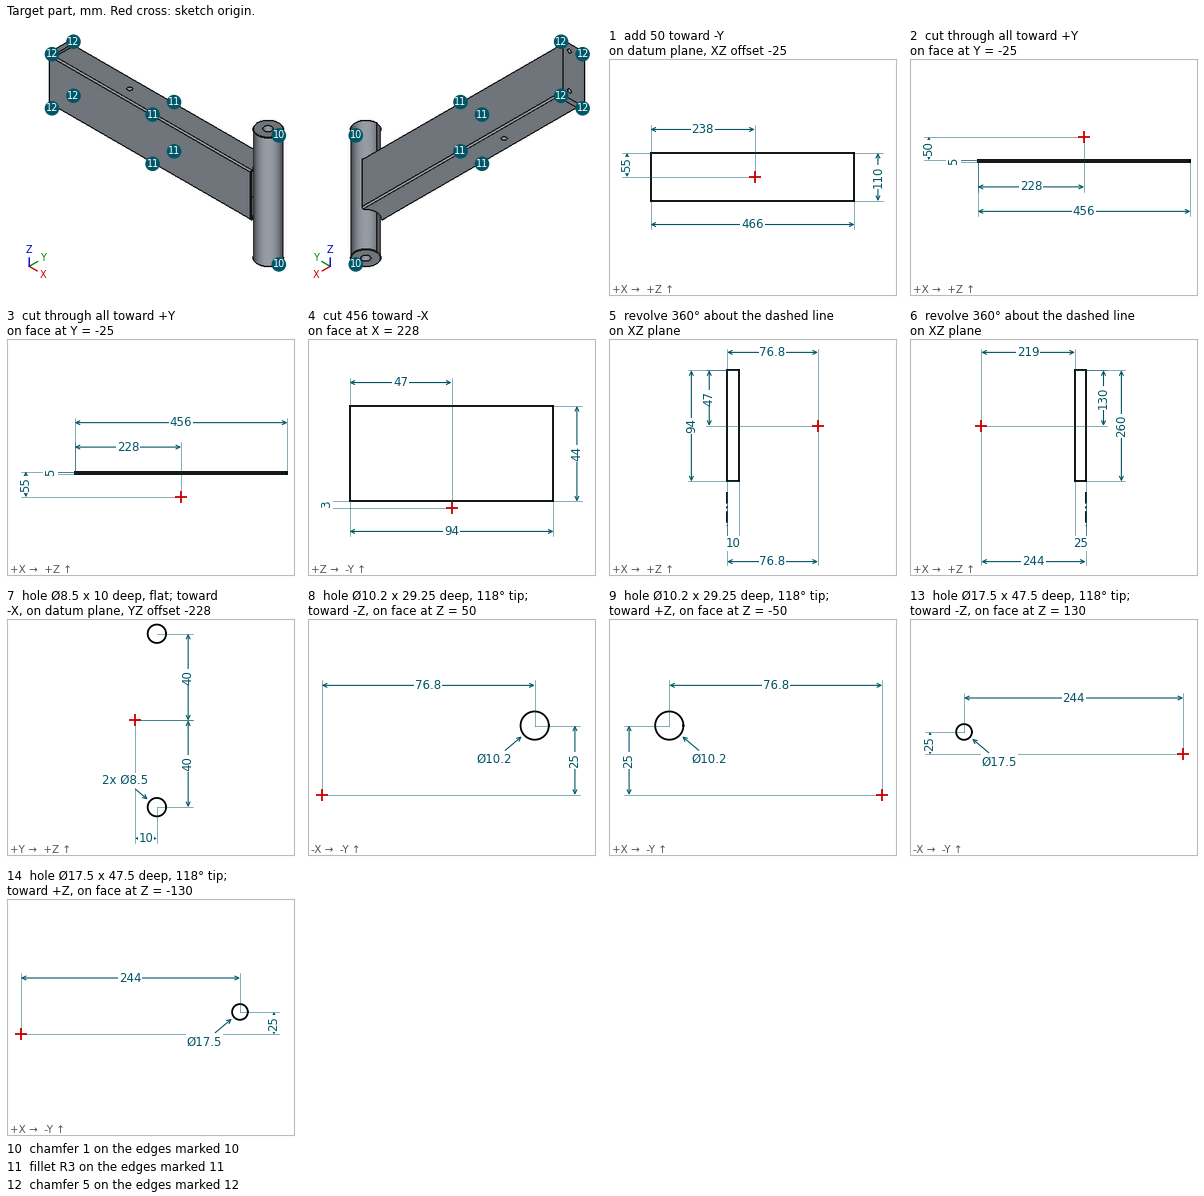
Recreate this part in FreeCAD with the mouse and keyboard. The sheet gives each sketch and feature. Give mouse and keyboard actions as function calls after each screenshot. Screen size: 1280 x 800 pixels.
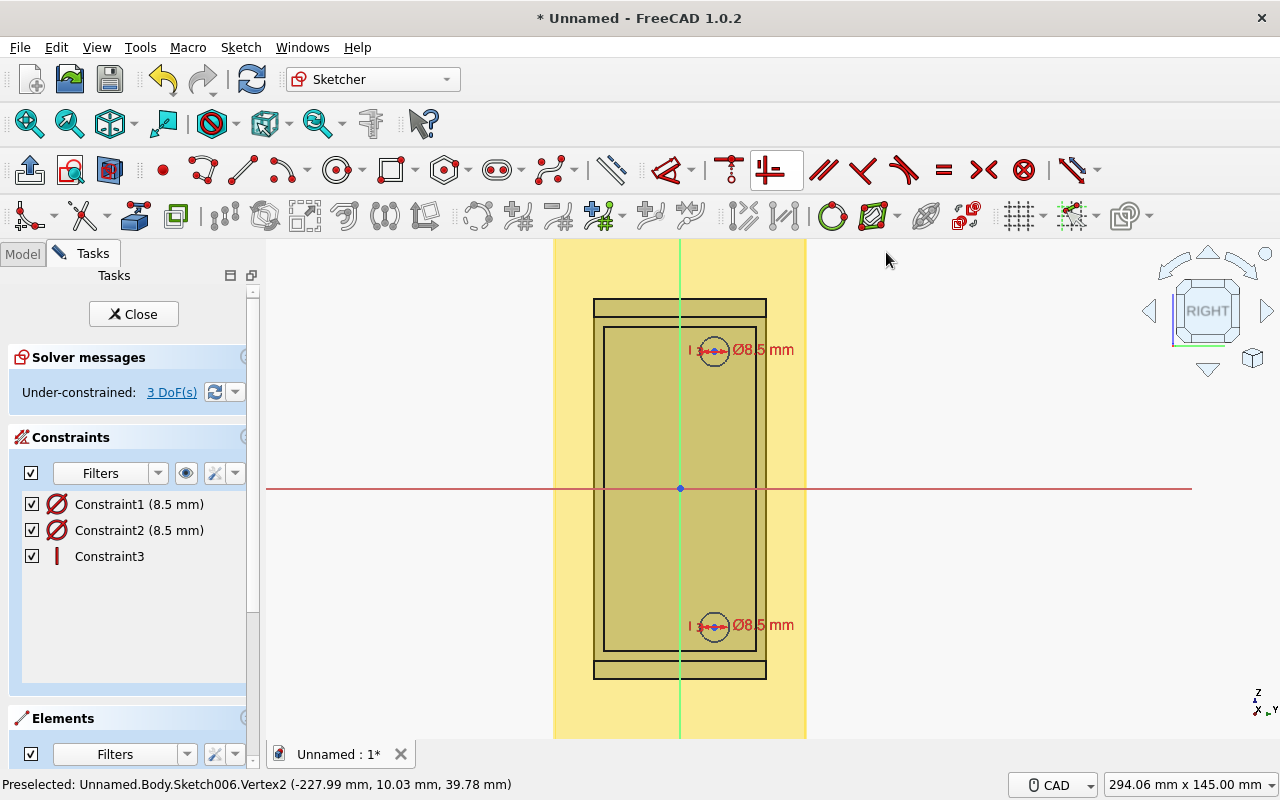
click(666, 170)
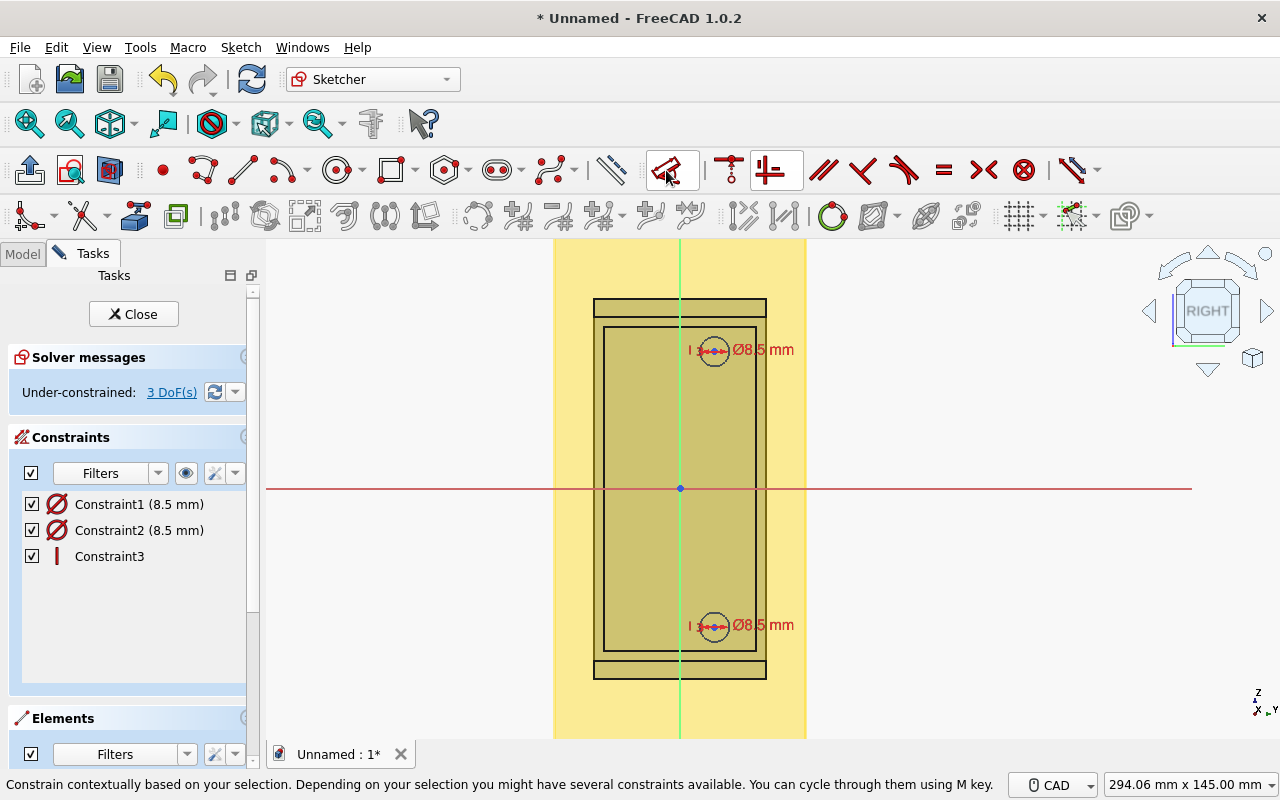
click(715, 627)
click(697, 661)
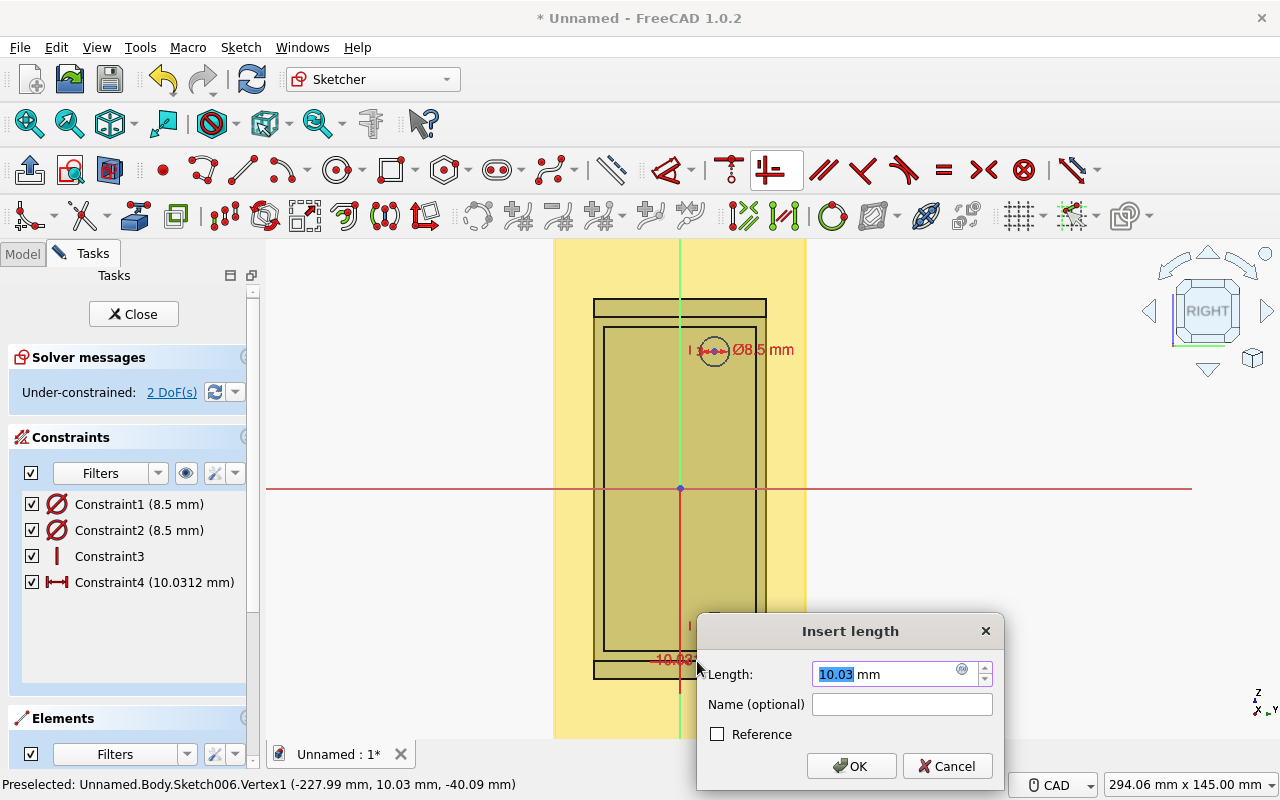
text(10)
key(Return)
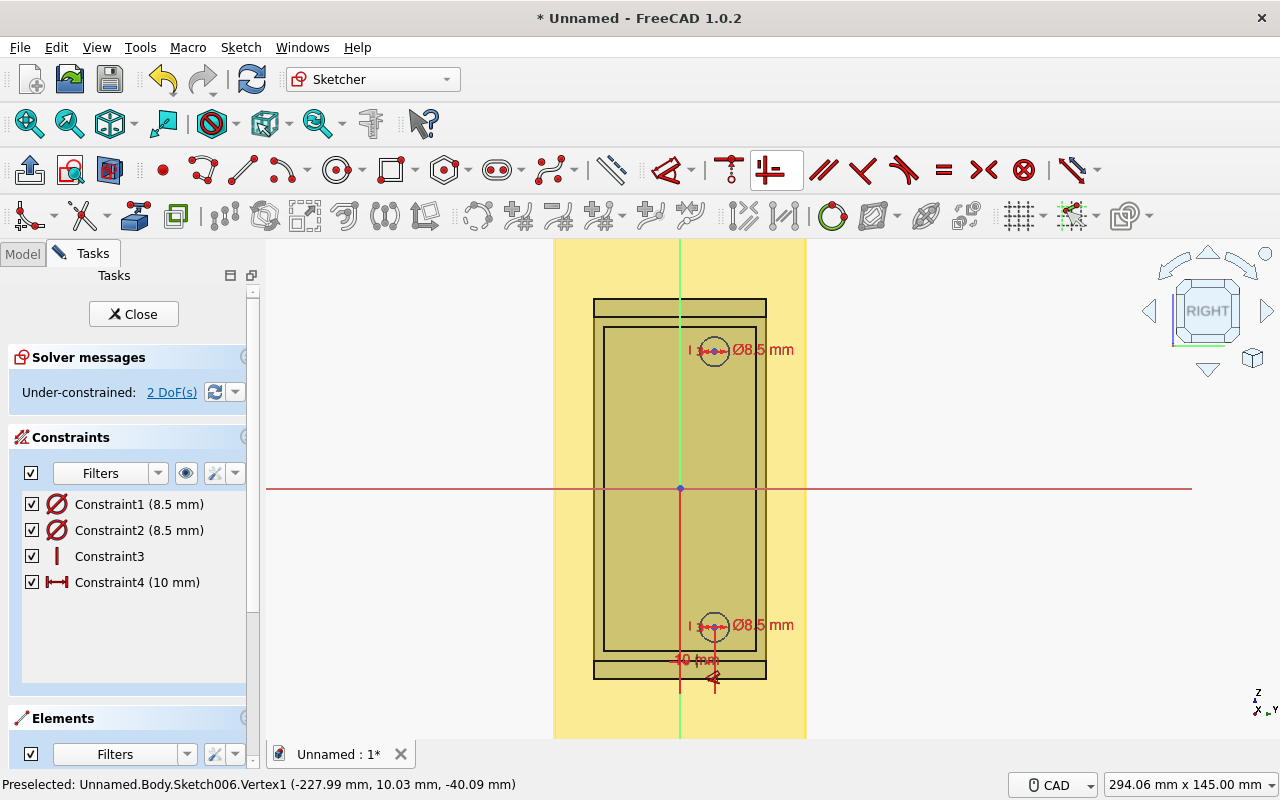
click(715, 627)
click(646, 558)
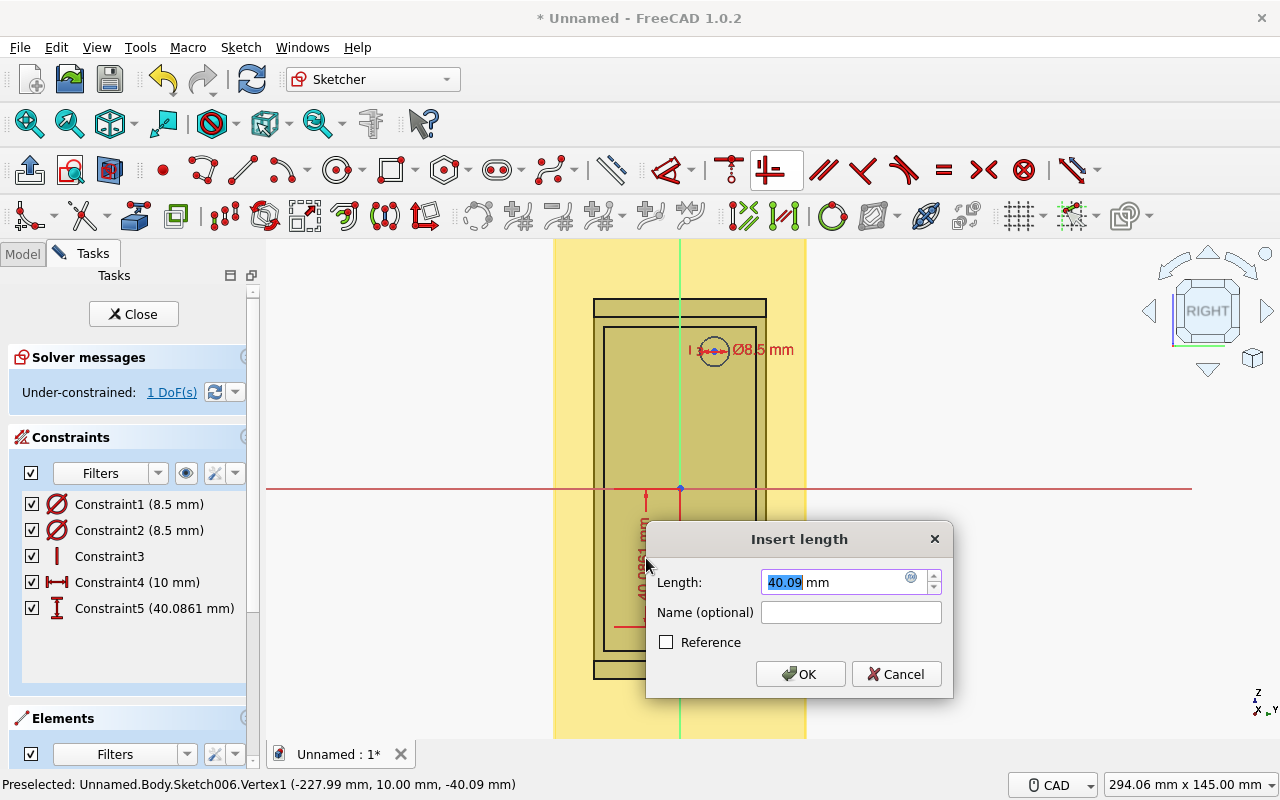
text(40)
key(Return)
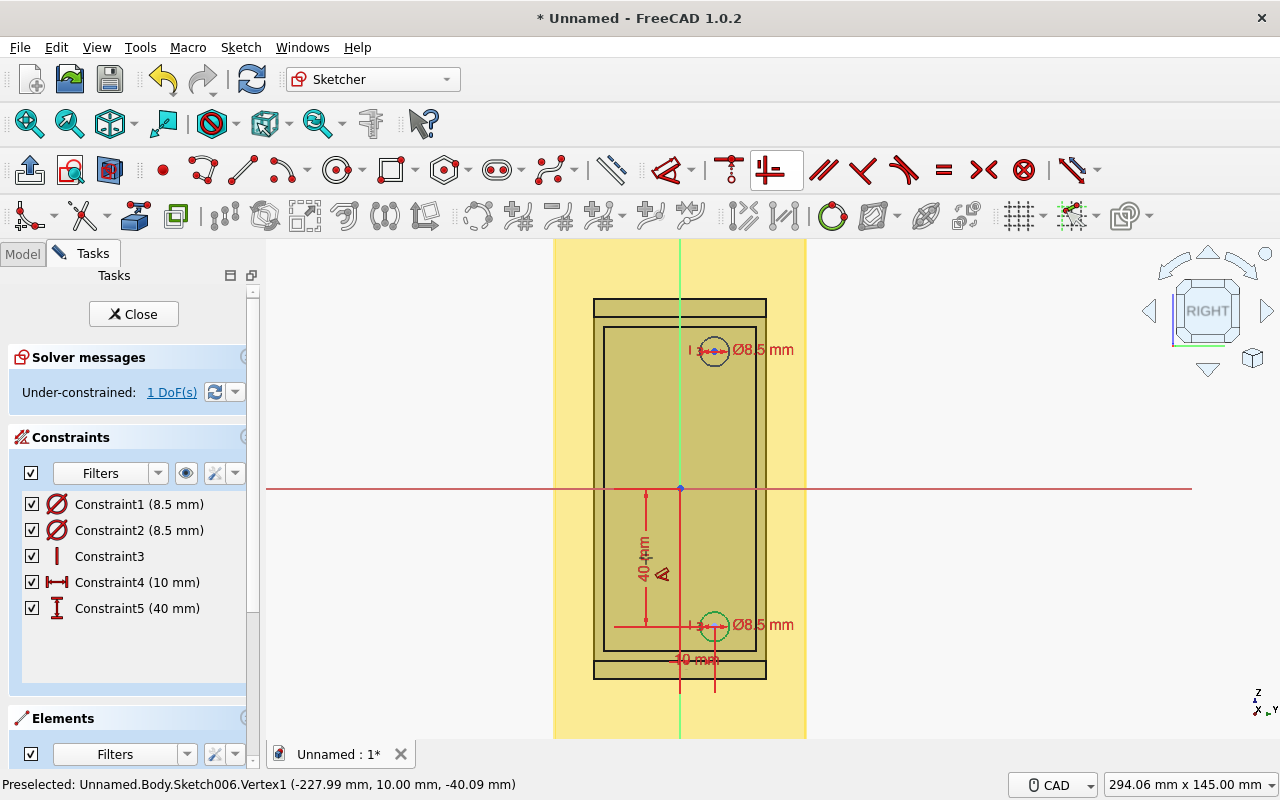
click(715, 352)
click(646, 420)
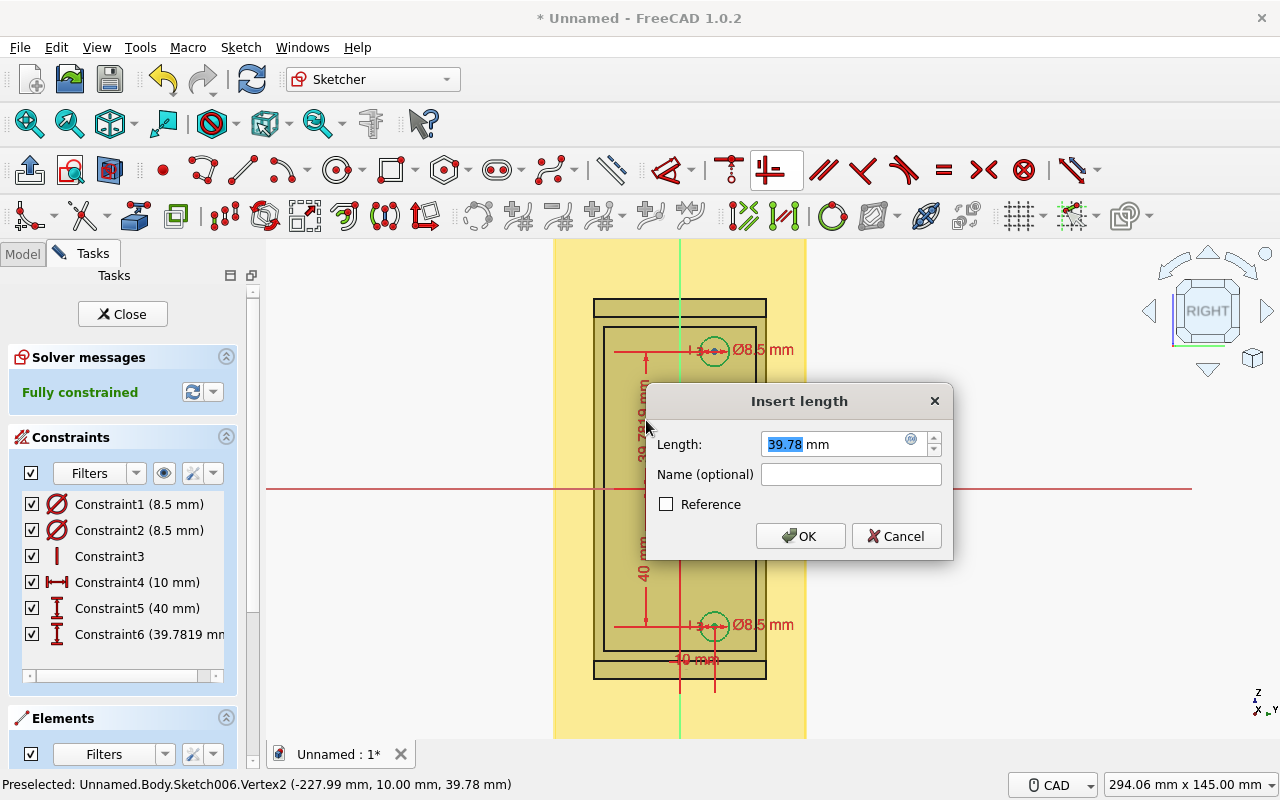
text(40)
key(Return)
key(Escape)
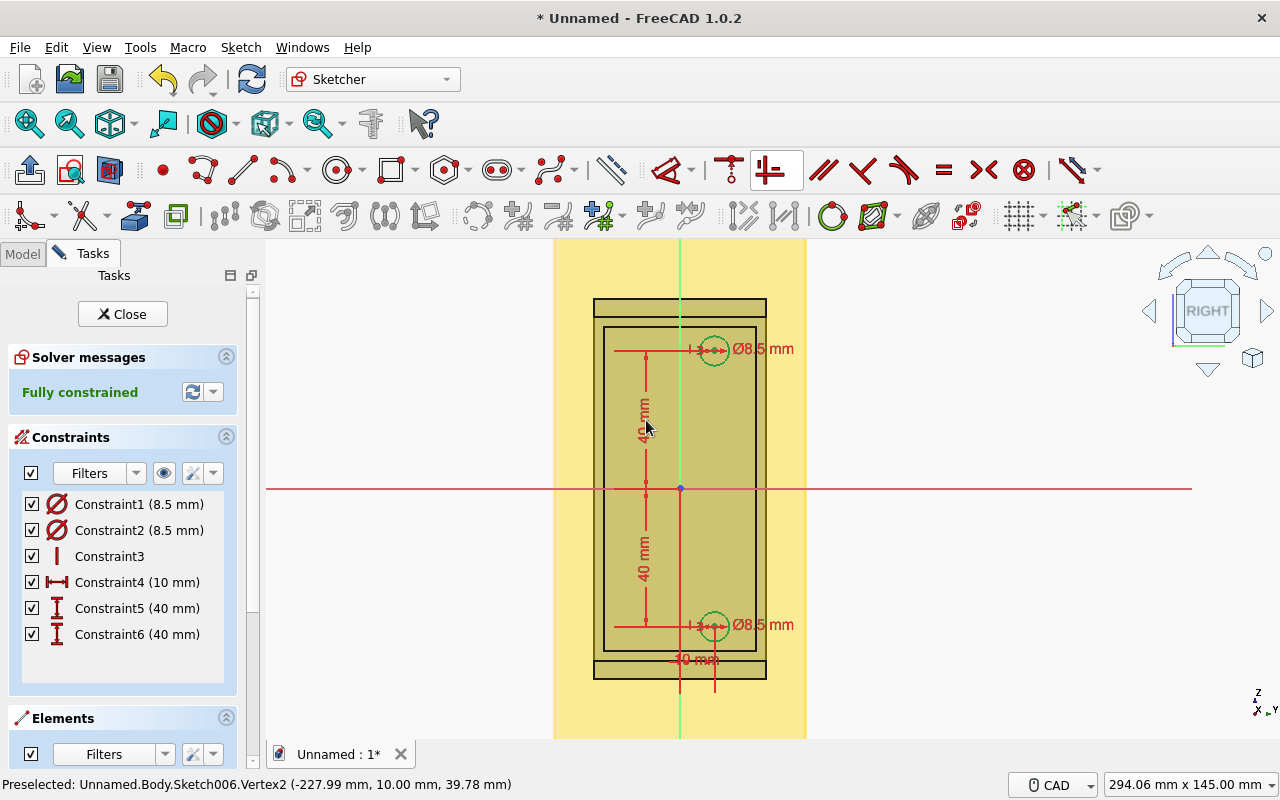
click(123, 314)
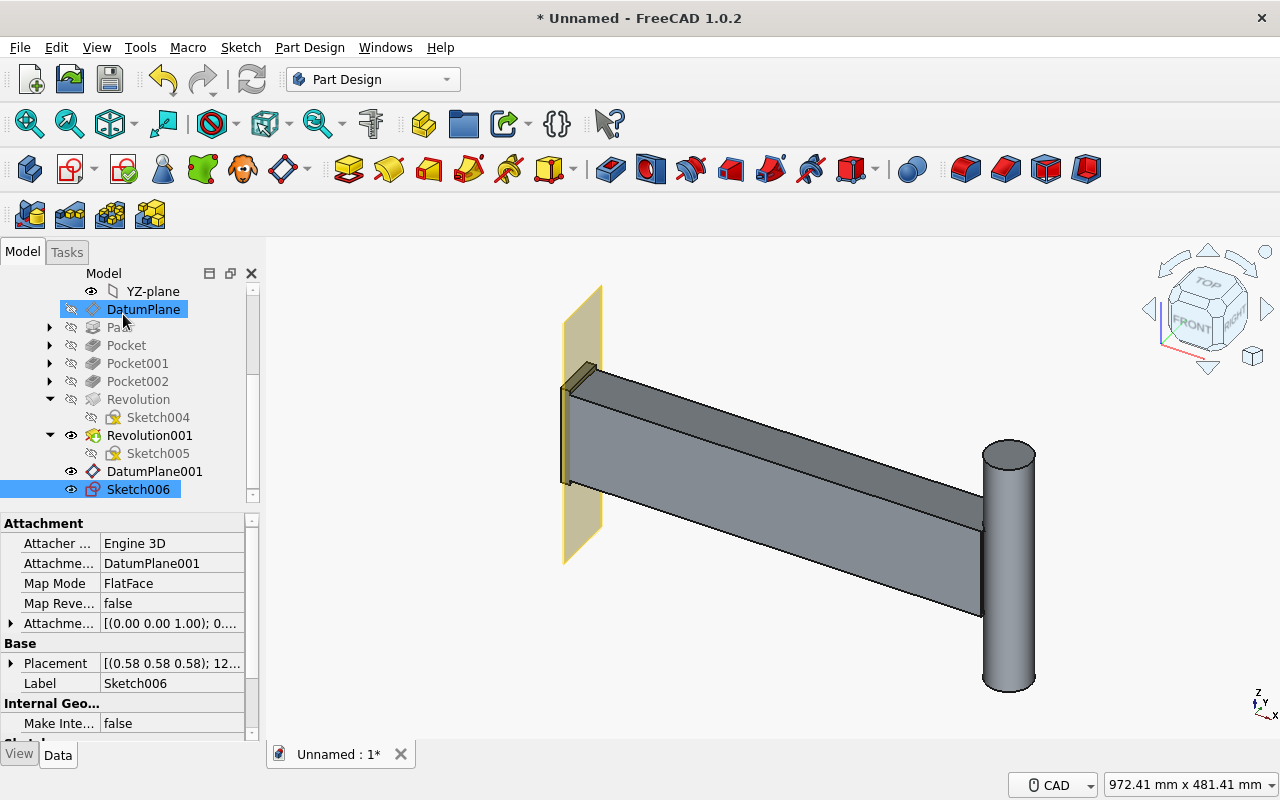
click(652, 170)